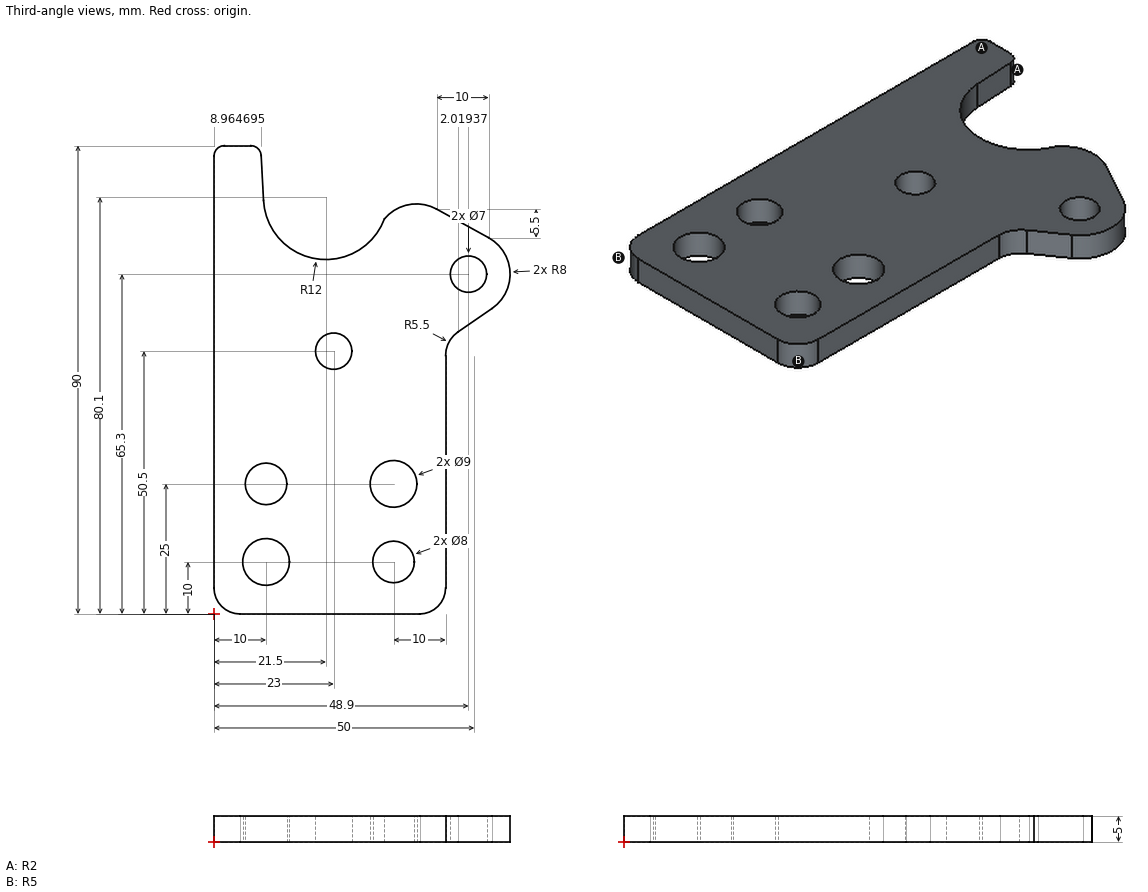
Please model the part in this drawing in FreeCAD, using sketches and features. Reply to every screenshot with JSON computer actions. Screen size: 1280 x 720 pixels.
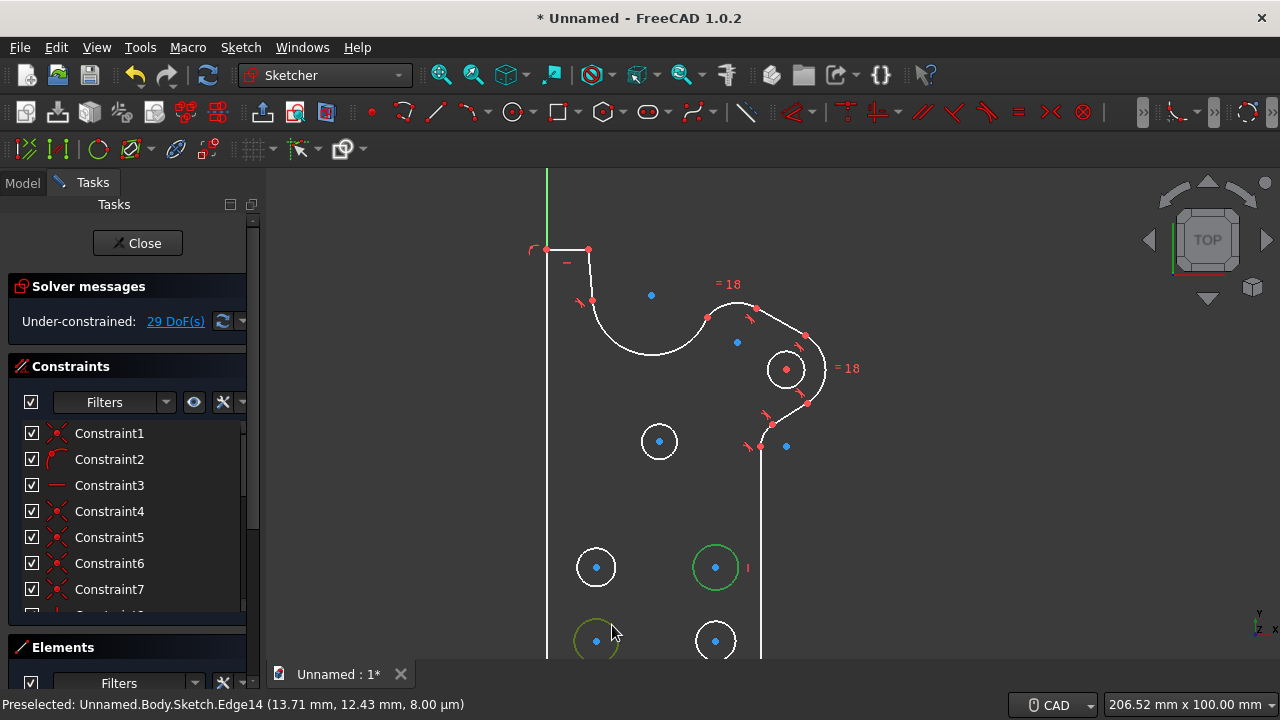
{"action": "key", "text": "e"}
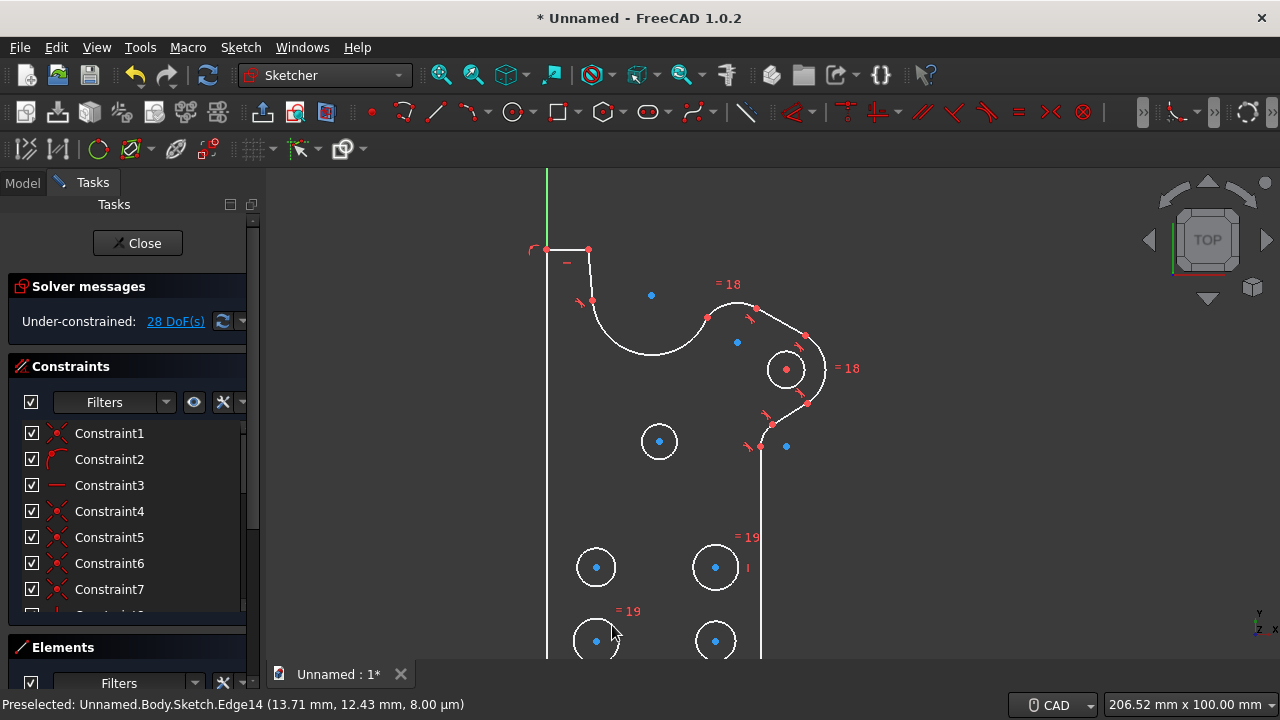
{"action": "left_click", "coordinate": [730, 627]}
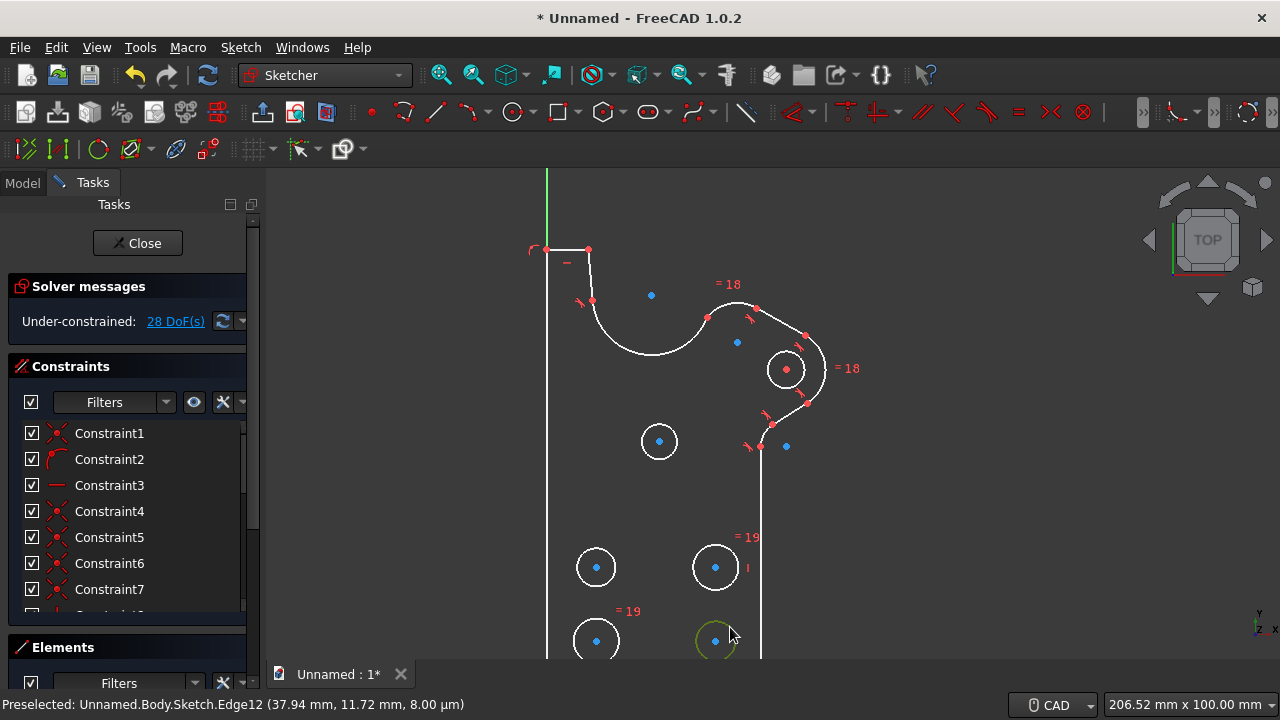
{"action": "left_click", "coordinate": [610, 554]}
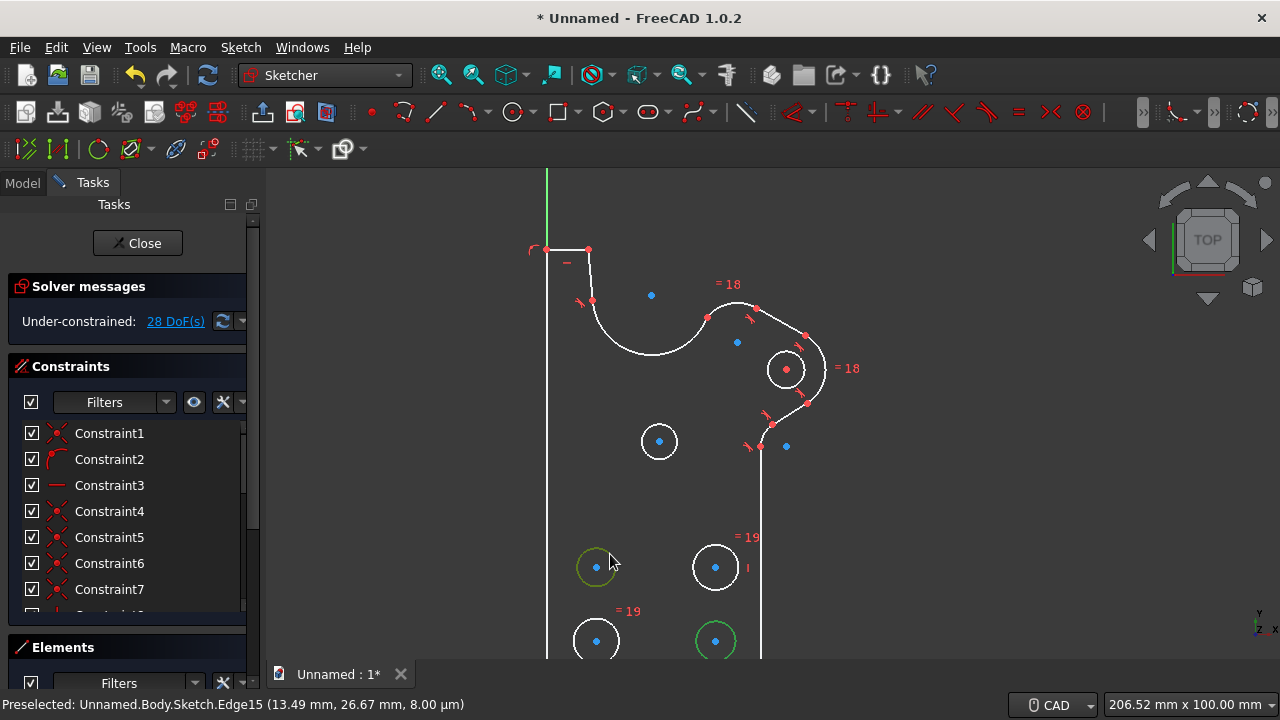
{"action": "left_click", "coordinate": [1020, 112]}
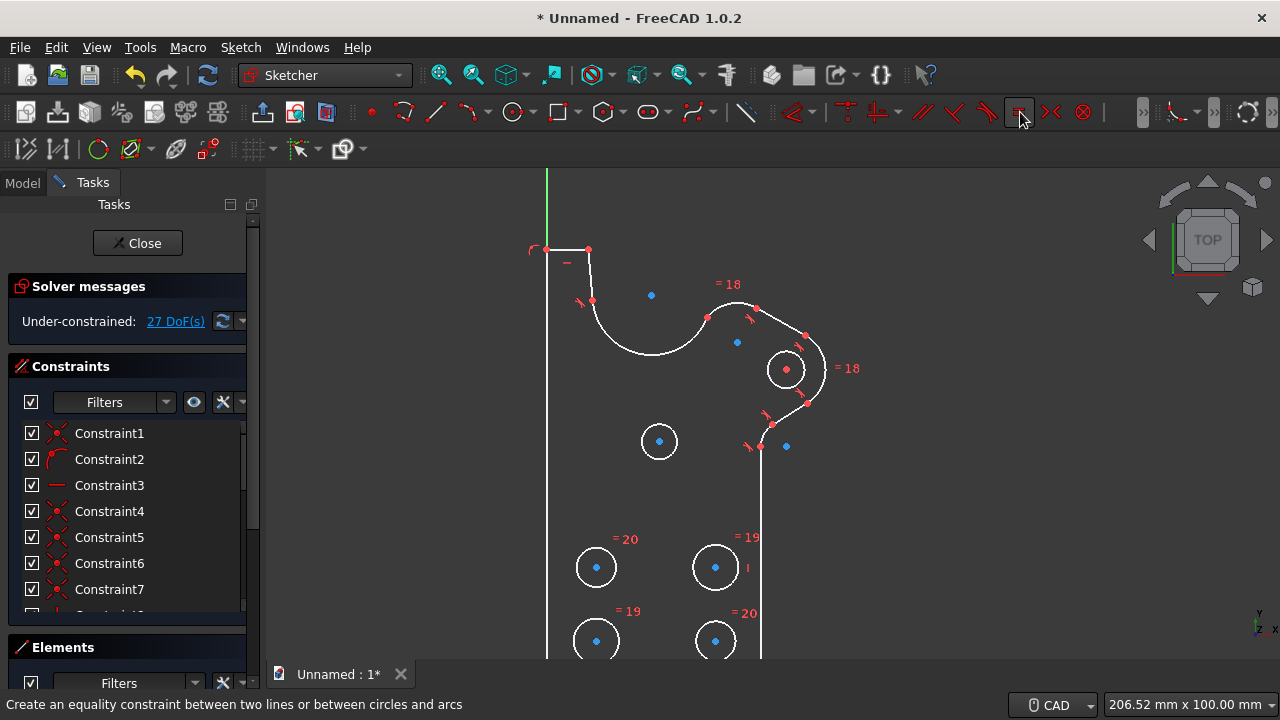
{"action": "left_click", "coordinate": [799, 357]}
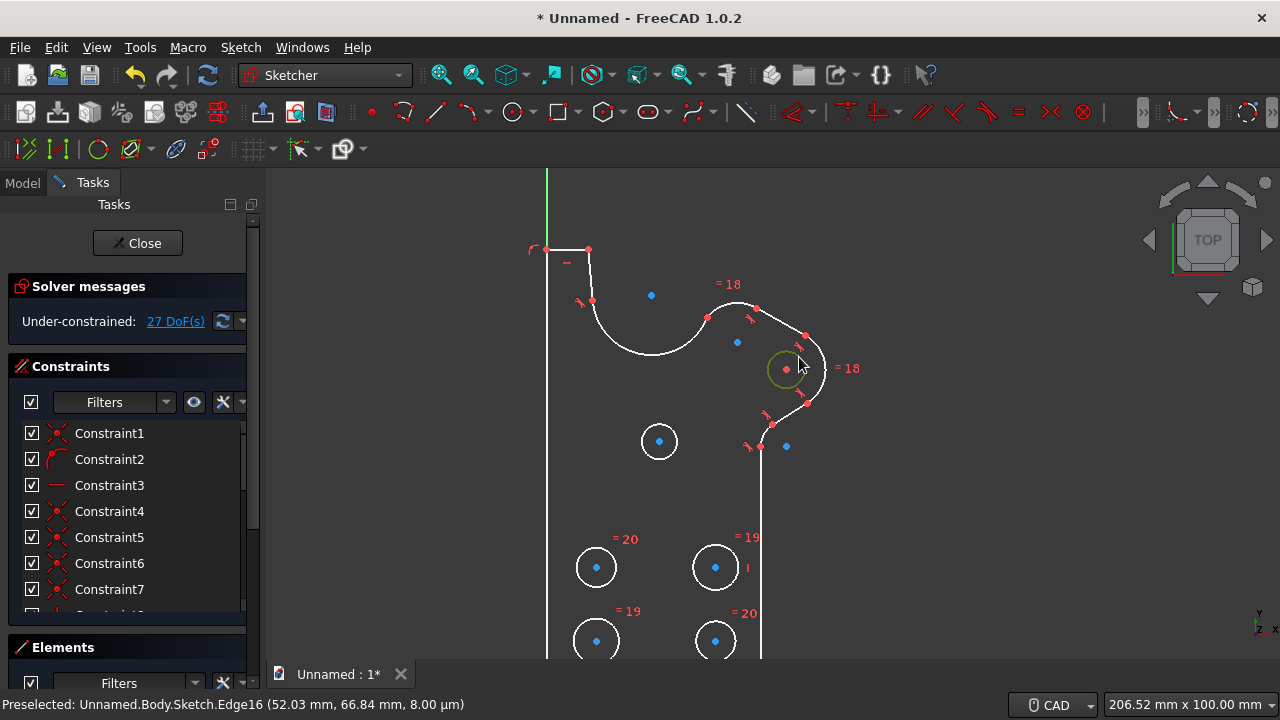
{"action": "left_click", "coordinate": [672, 429]}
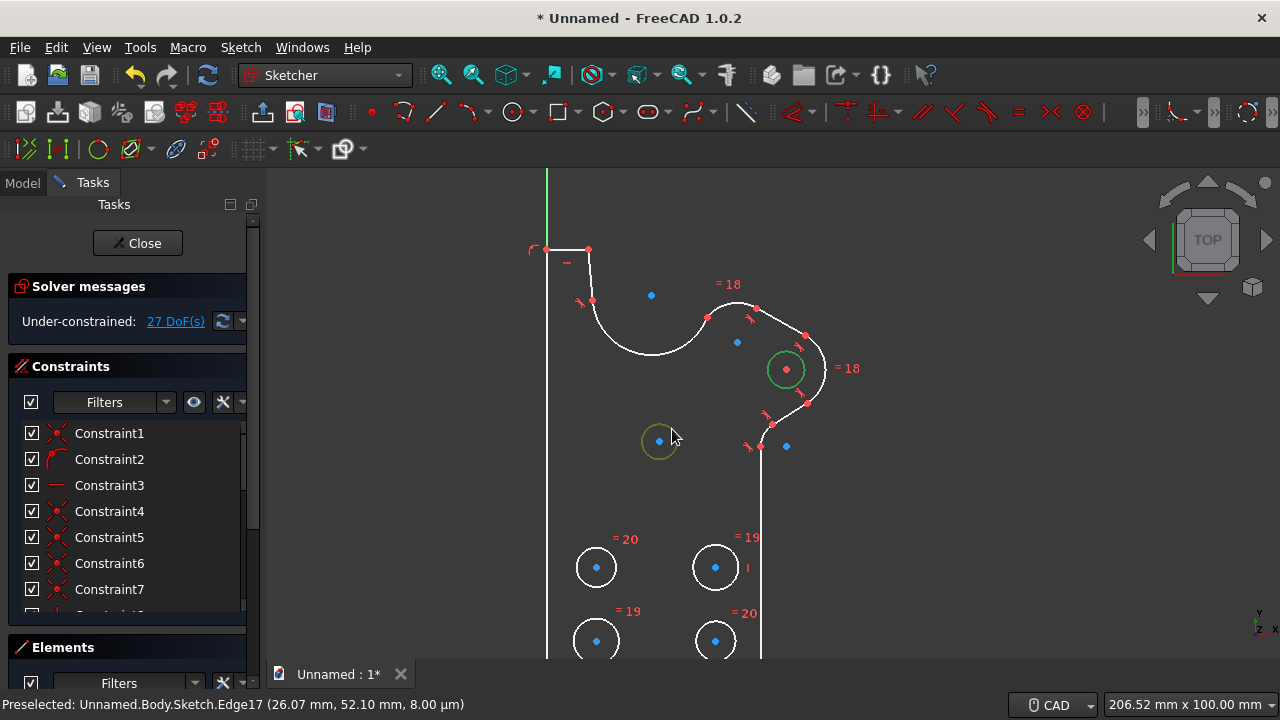
{"action": "key", "text": "e"}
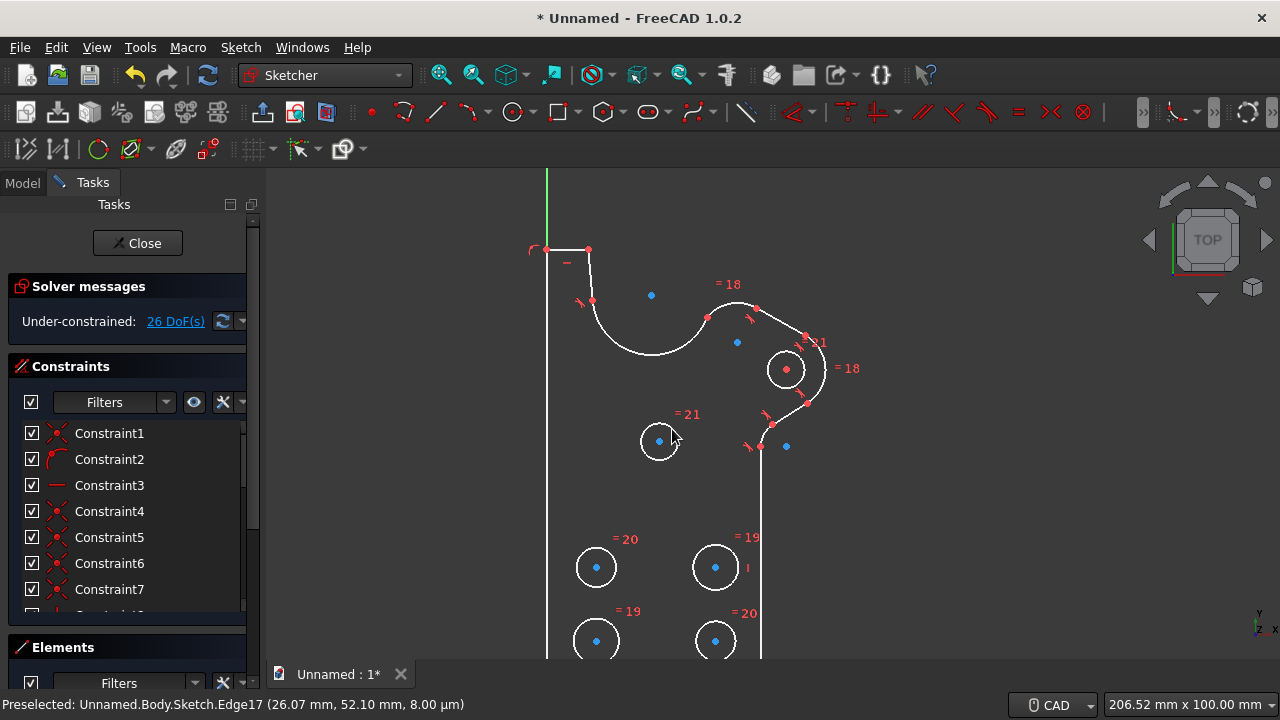
{"action": "left_click", "coordinate": [792, 112]}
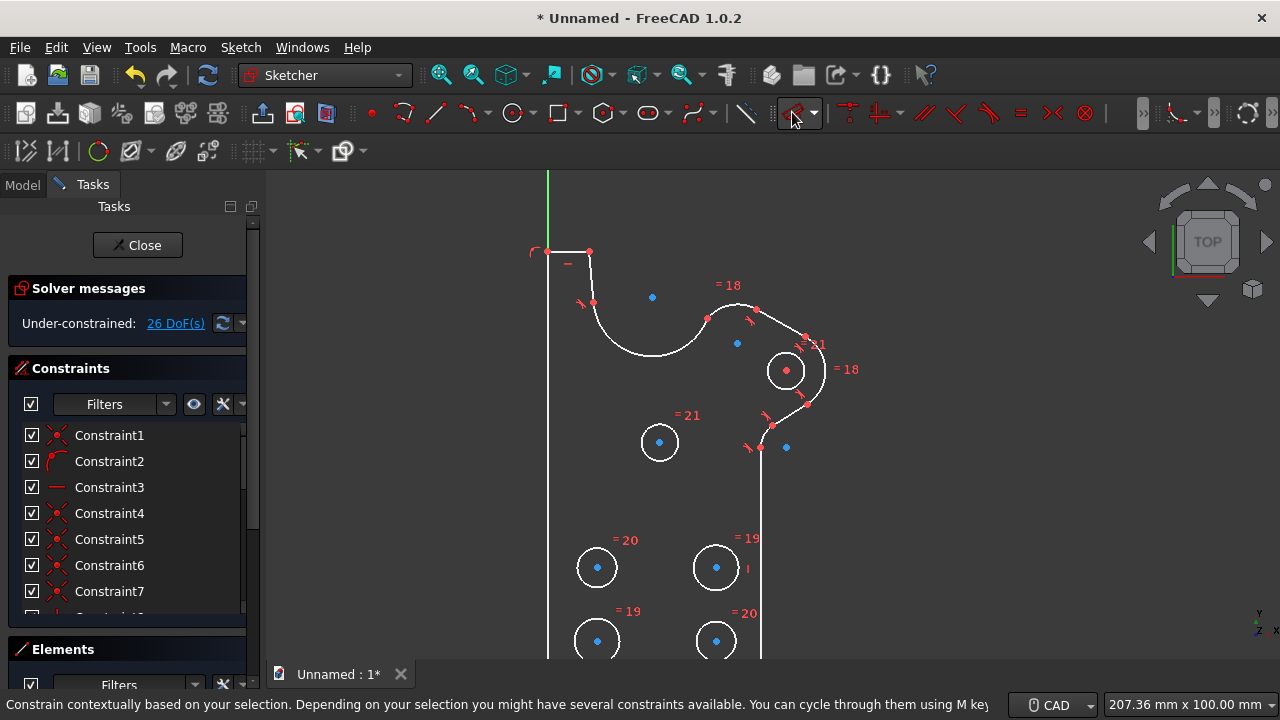
{"action": "scroll", "coordinate": [764, 435], "scroll_direction": "up", "scroll_amount": 2}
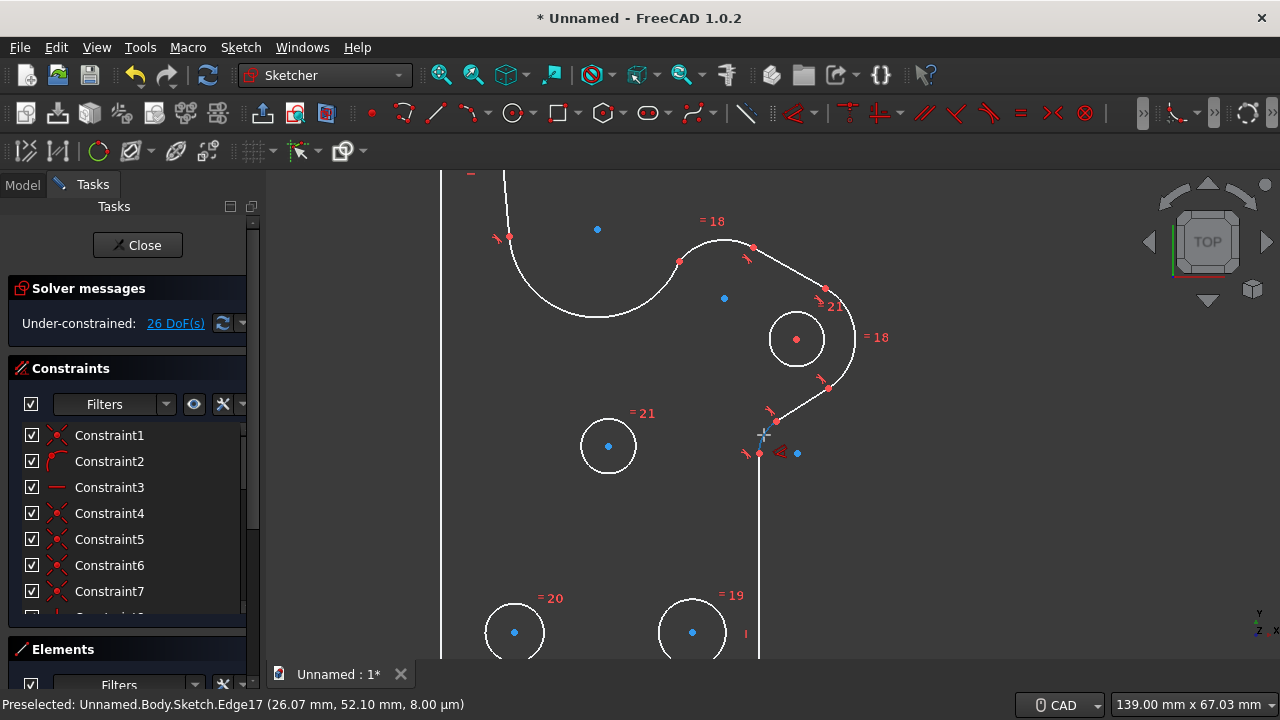
{"action": "left_click", "coordinate": [764, 435]}
{"action": "left_click", "coordinate": [736, 420]}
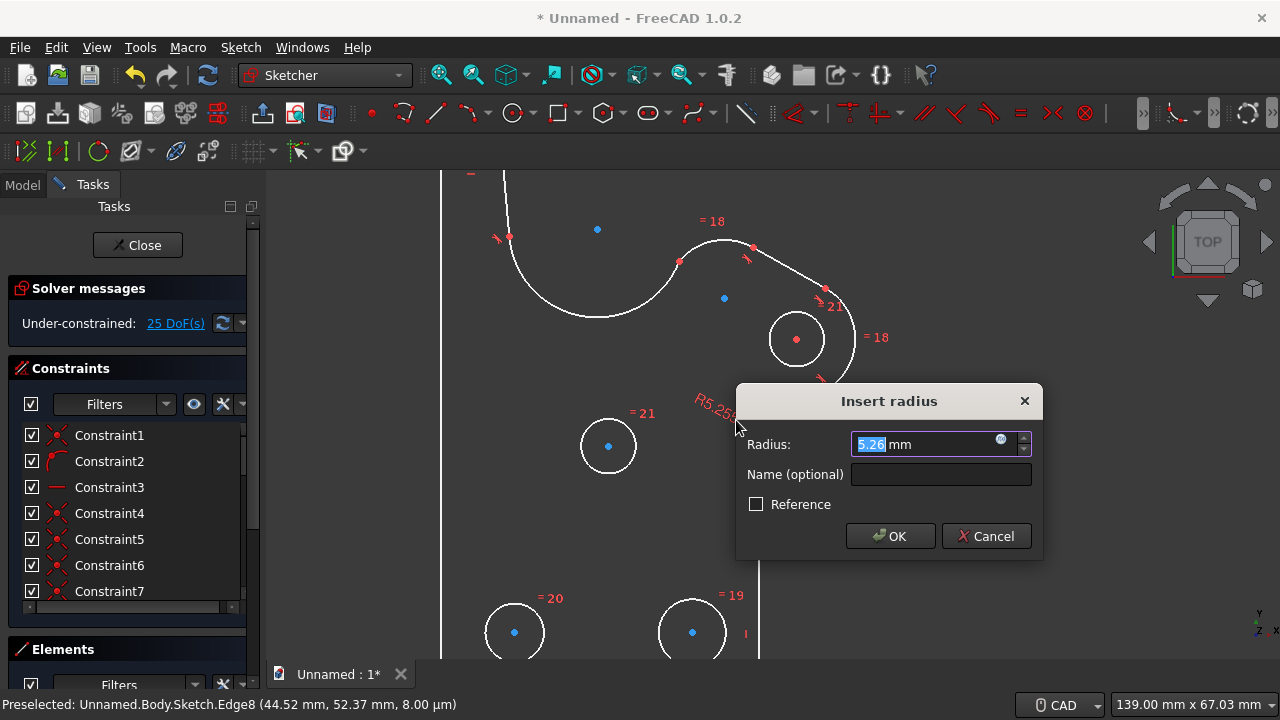
{"action": "type", "text": "5.5"}
{"action": "key", "text": "Return"}